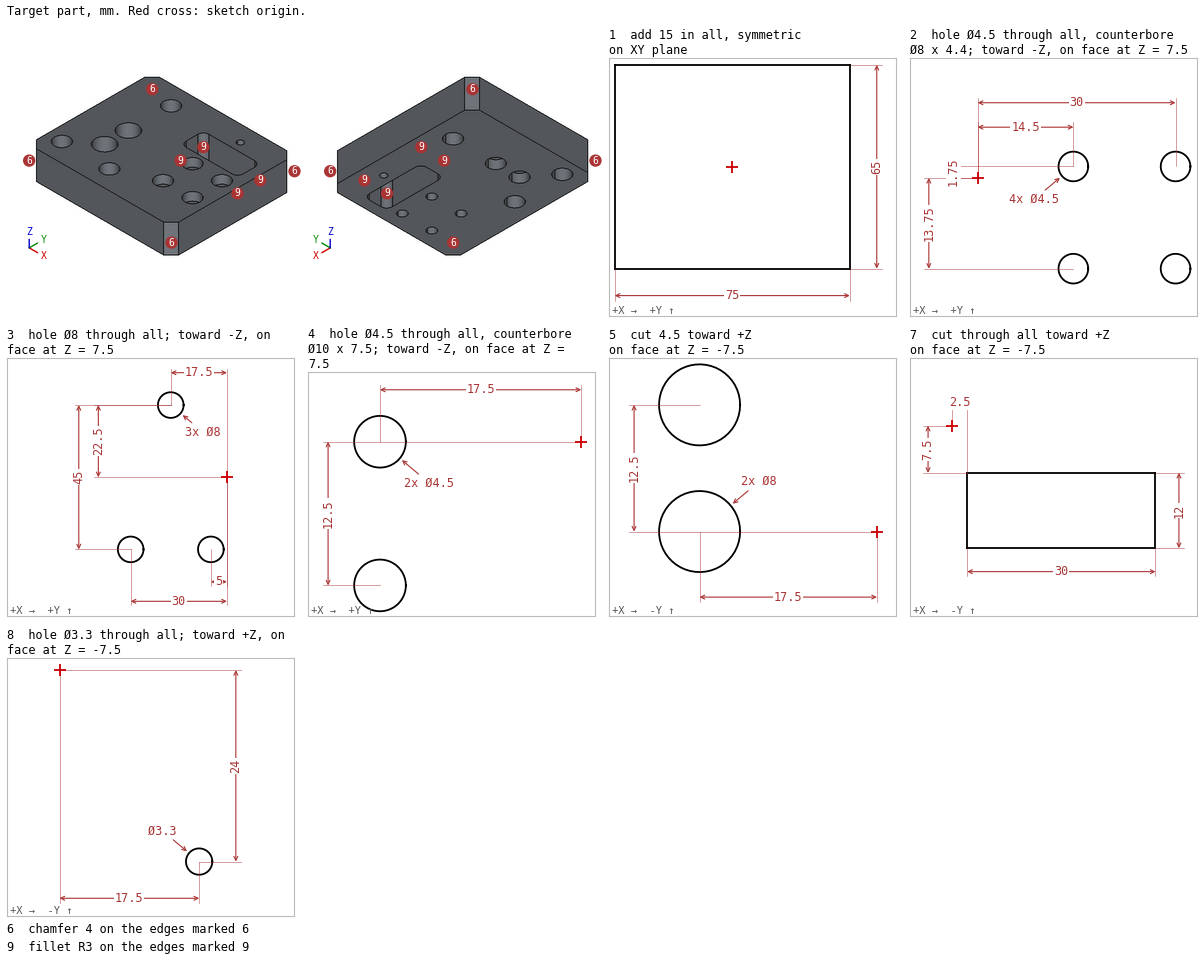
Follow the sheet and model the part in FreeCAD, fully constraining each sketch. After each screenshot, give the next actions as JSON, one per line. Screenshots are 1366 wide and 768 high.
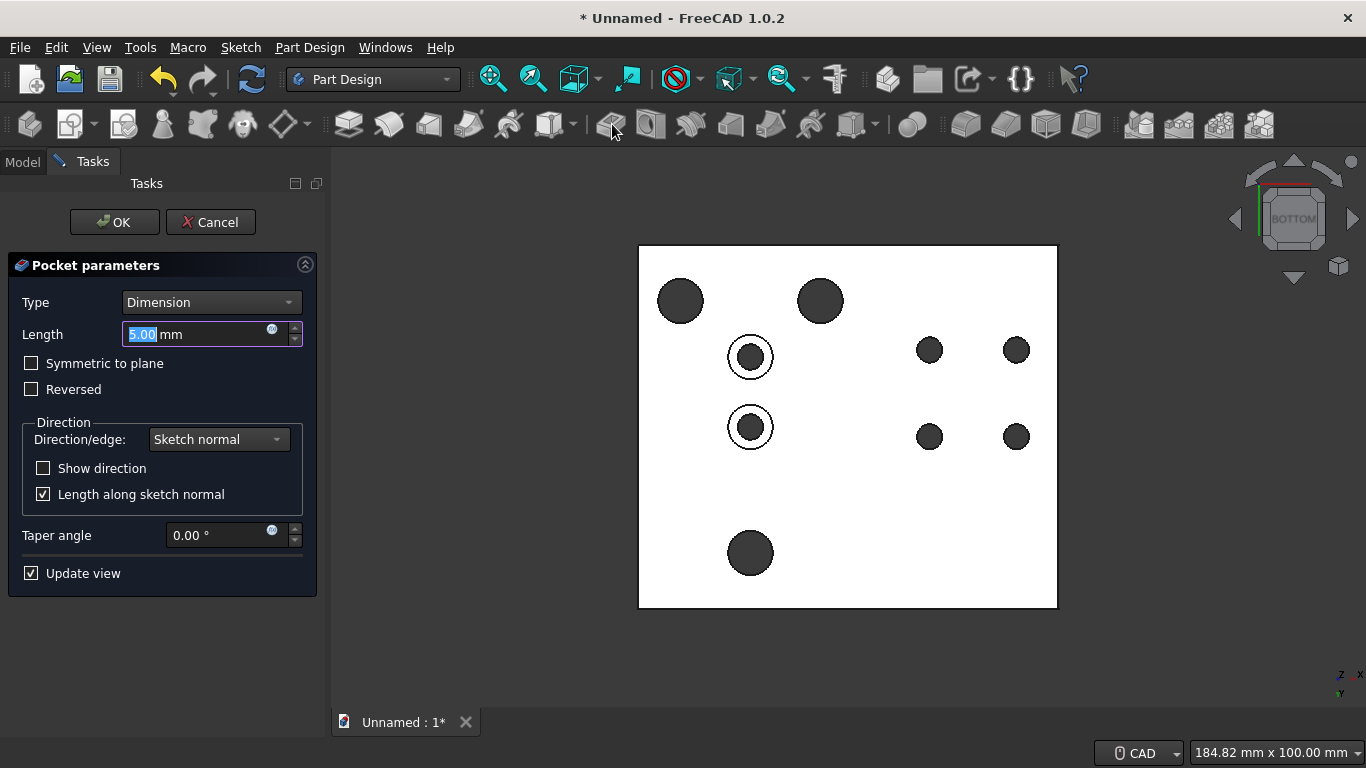
{"action": "type", "text": "4.5"}
{"action": "key", "text": "Tab"}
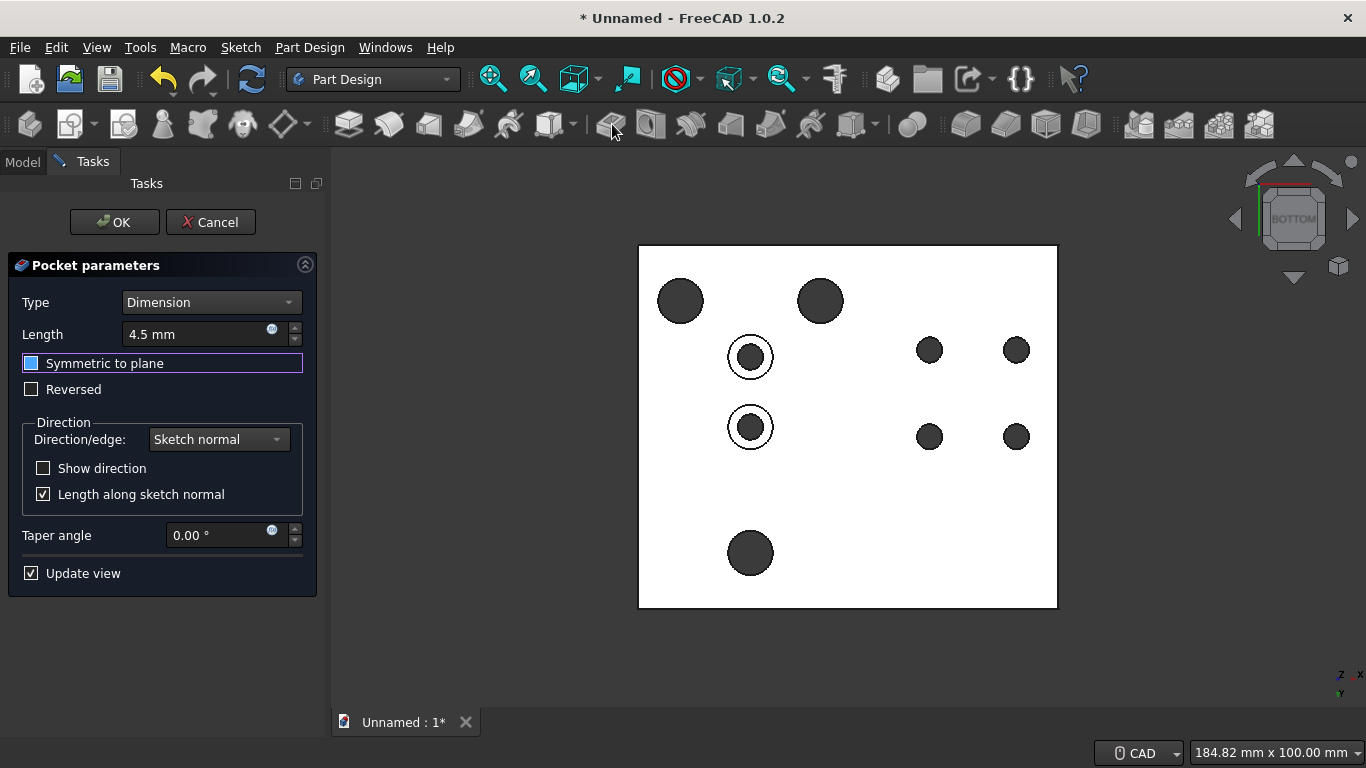
{"action": "left_click", "coordinate": [115, 222]}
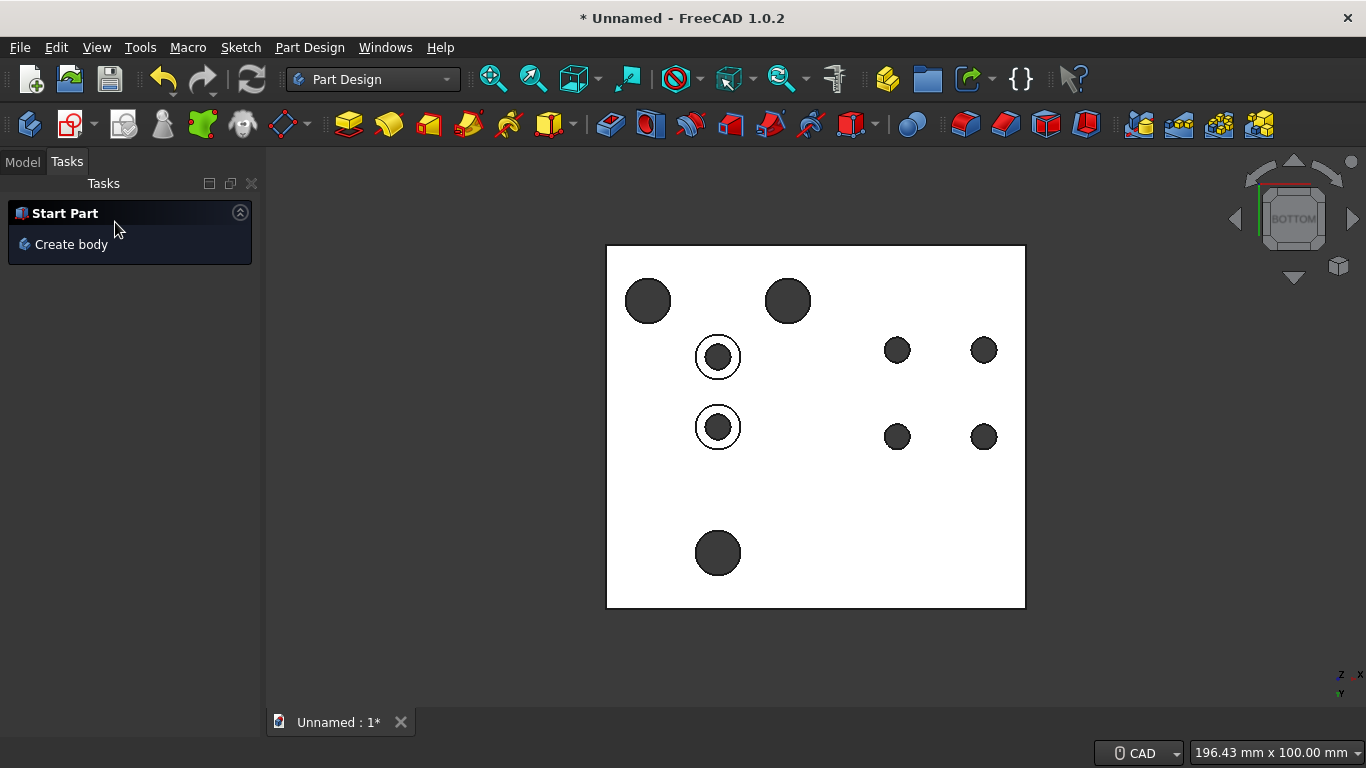
{"action": "key", "text": "0"}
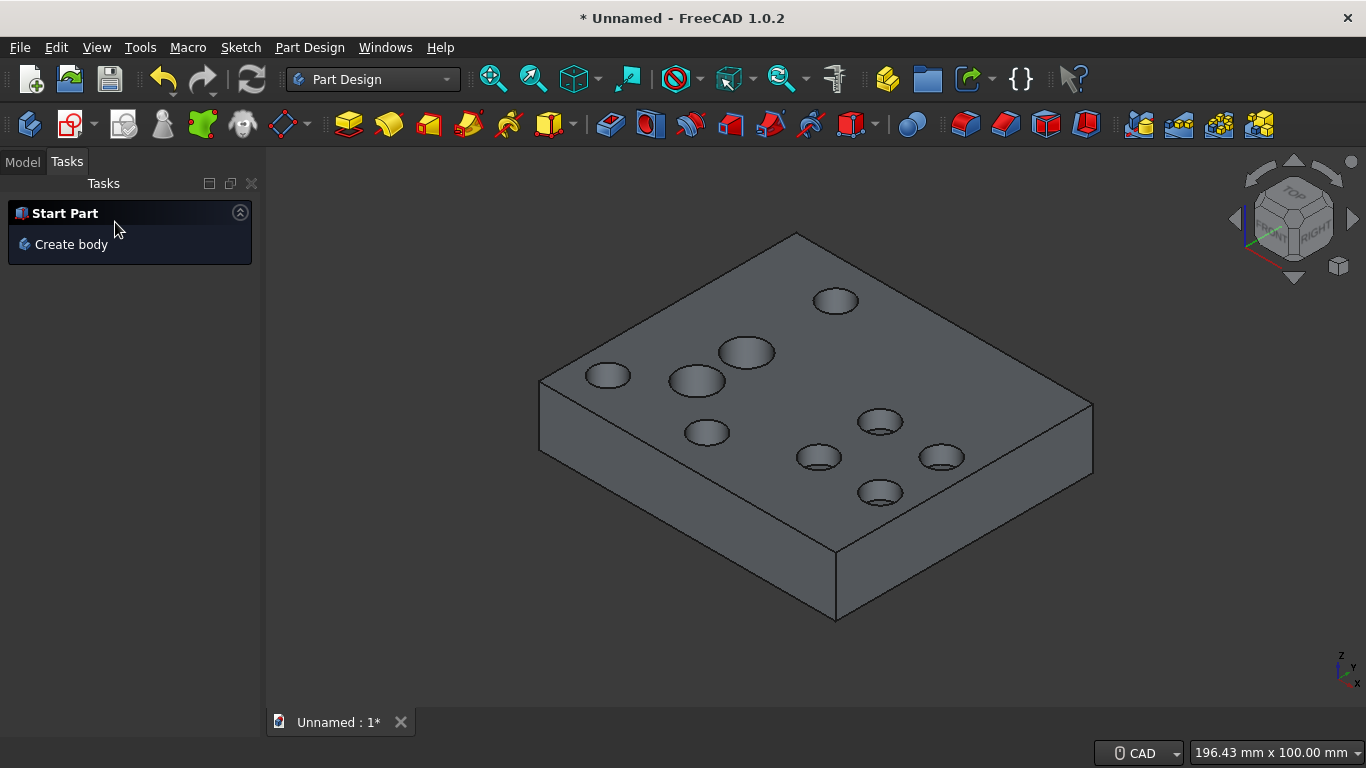
{"action": "left_click", "coordinate": [836, 586]}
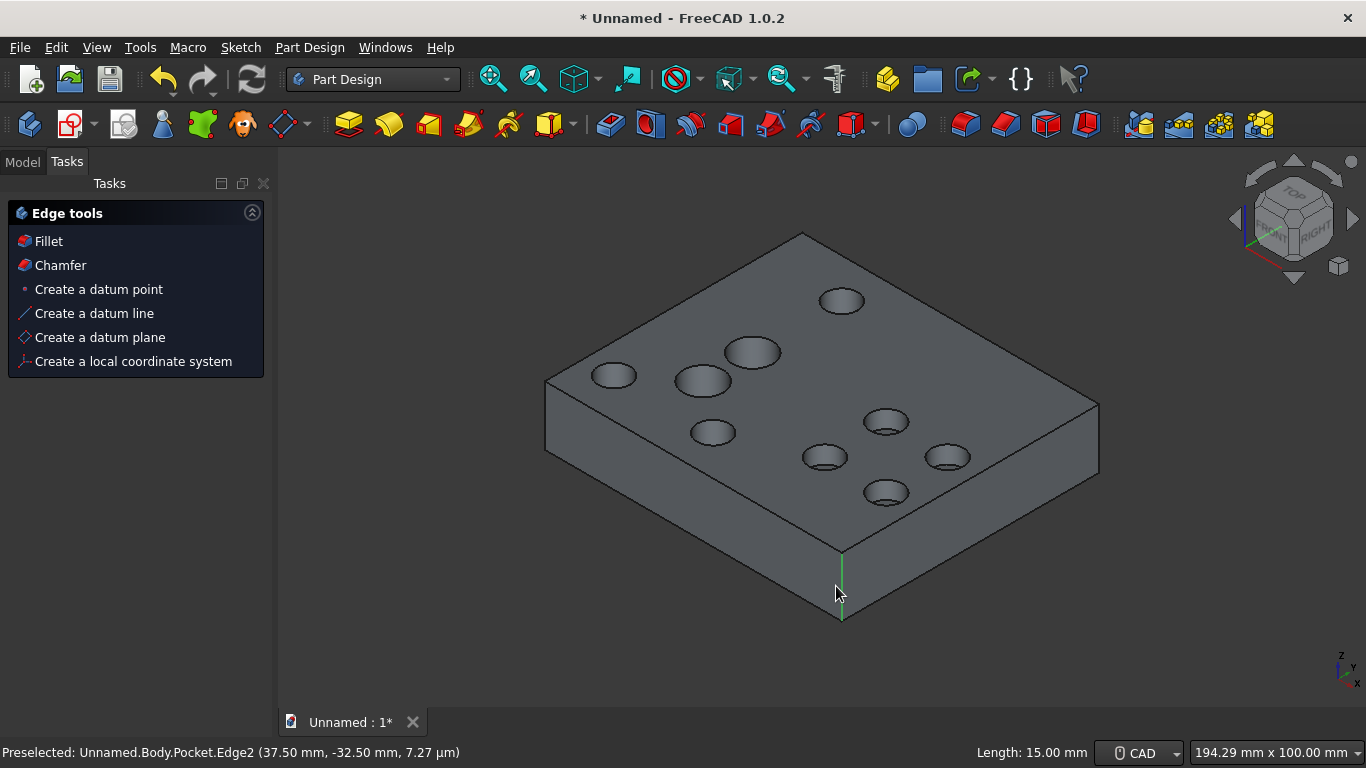
{"action": "key", "text": "2"}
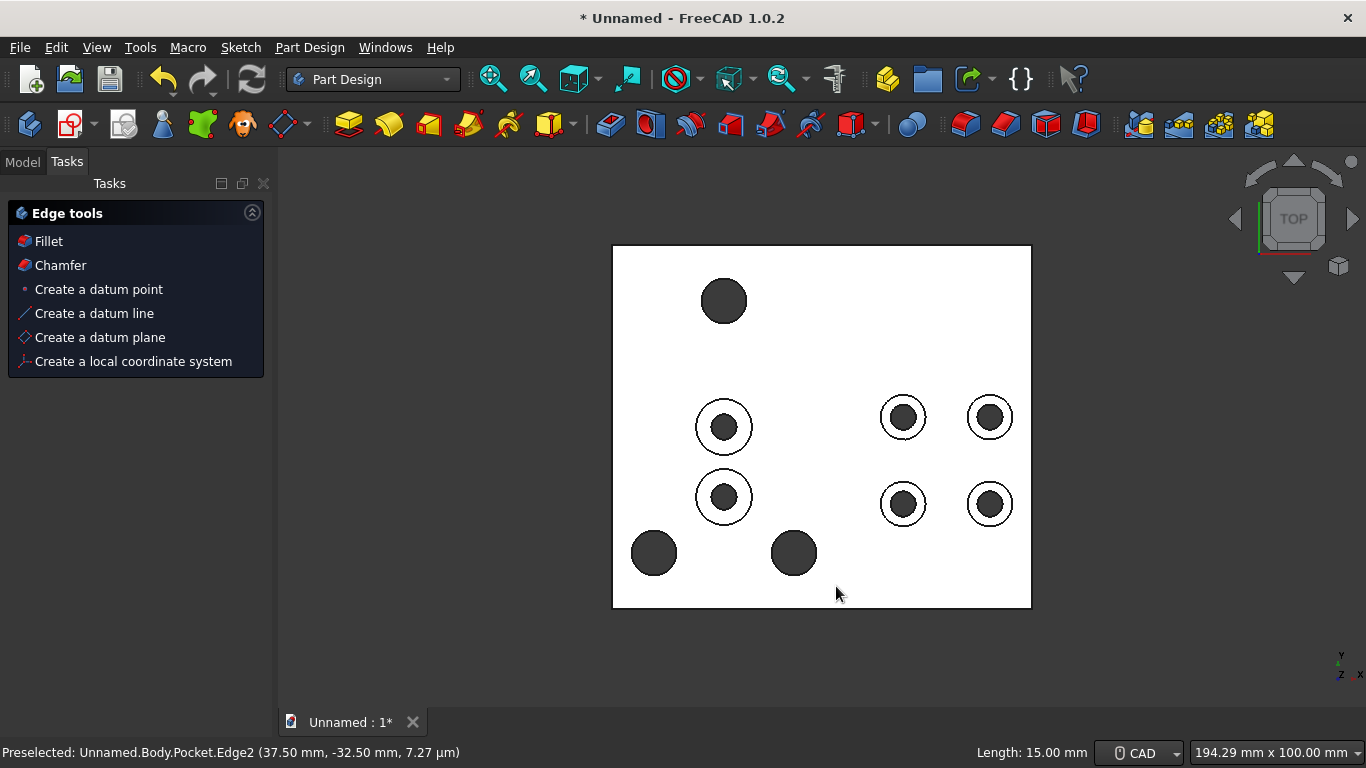
{"action": "key", "text": "1"}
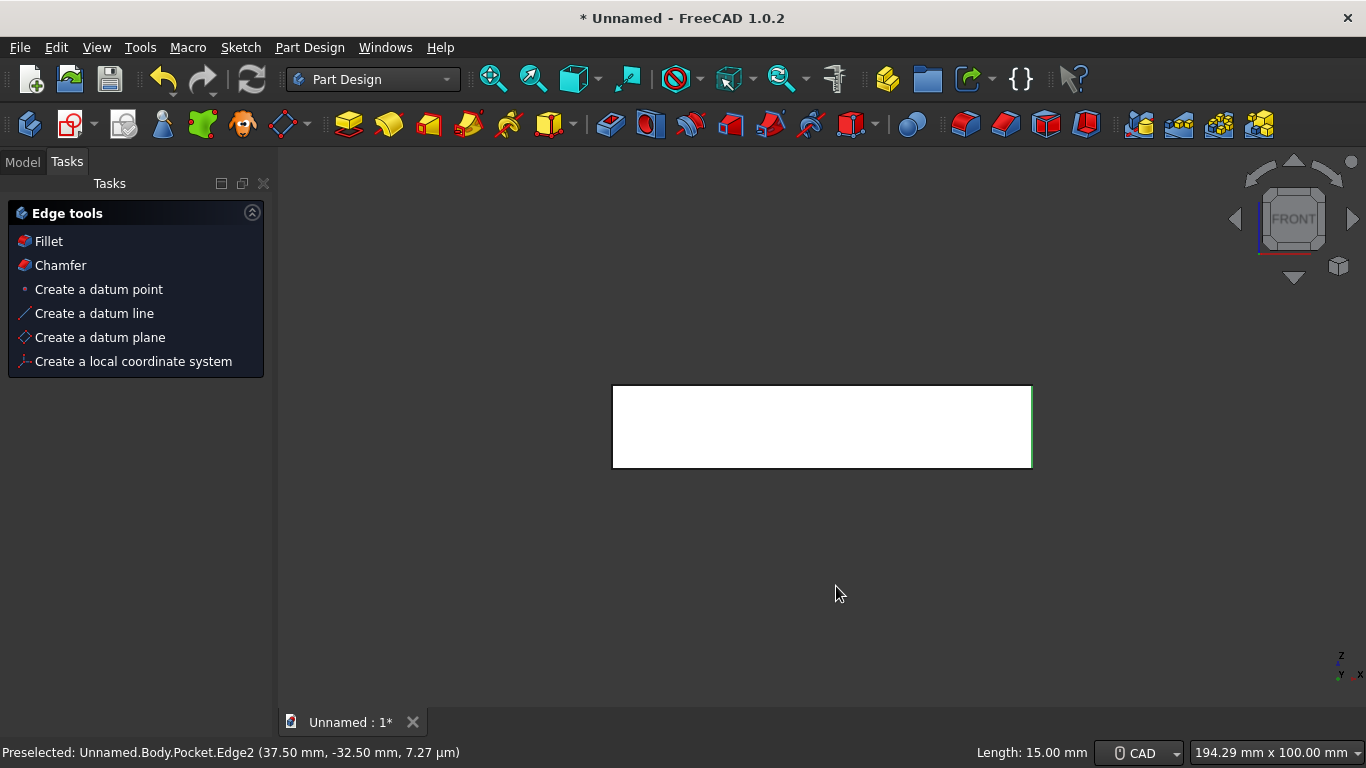
{"action": "key", "text": "v f"}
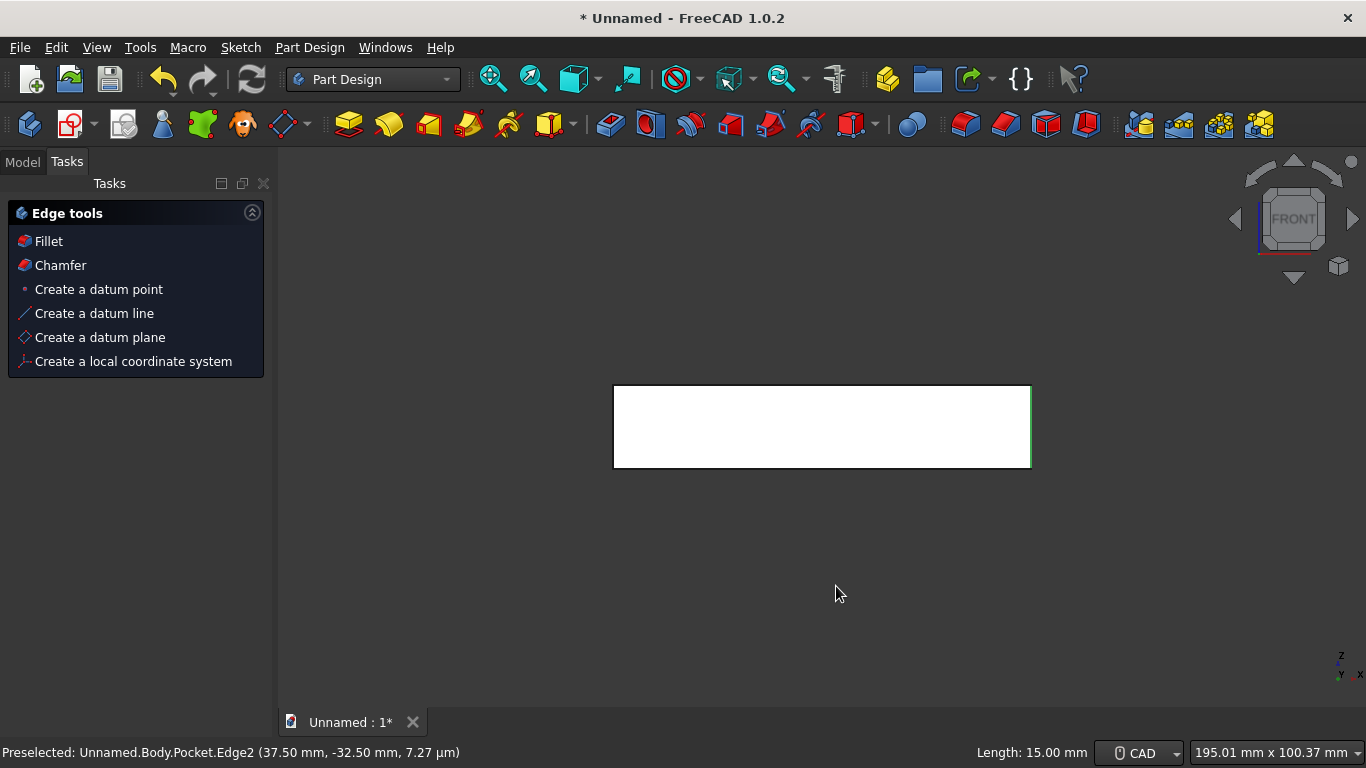
{"action": "left_click", "coordinate": [613, 426], "text": "ctrl"}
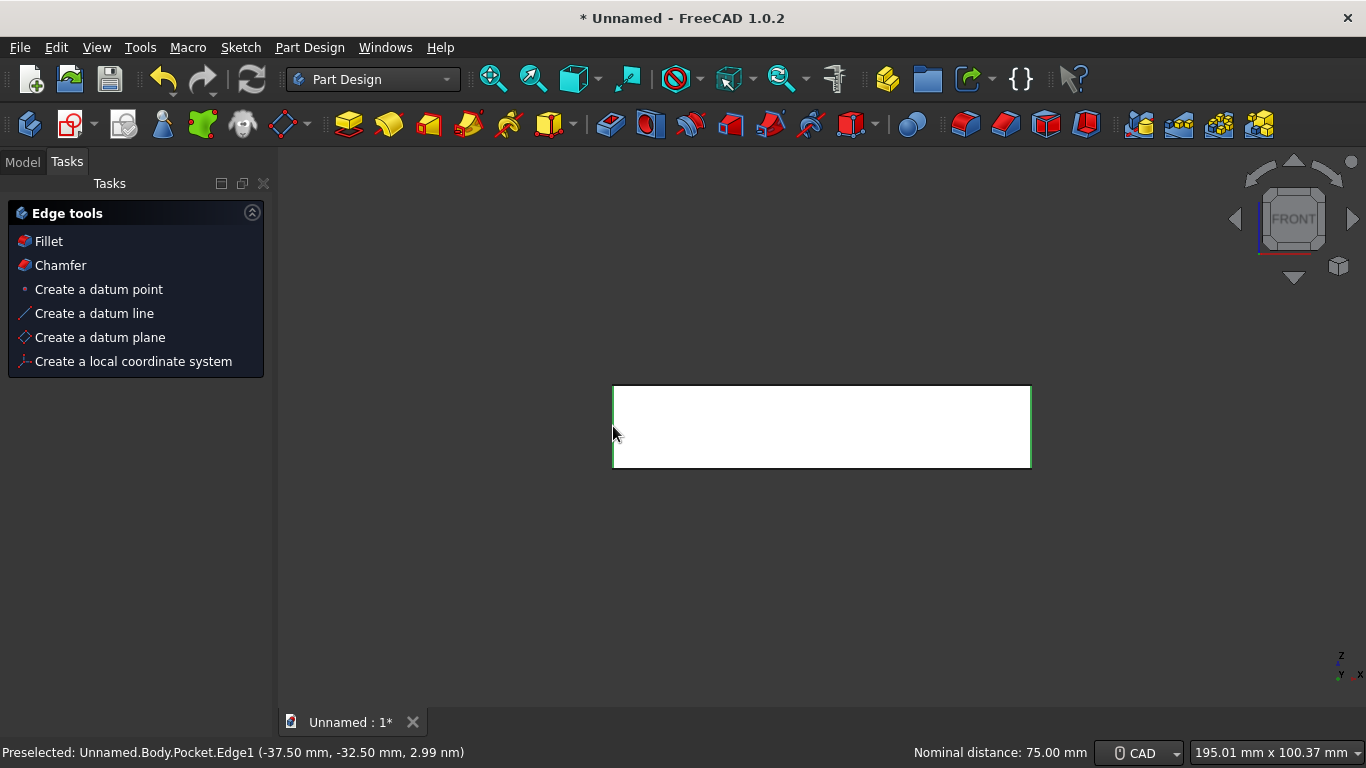
{"action": "key", "text": "3"}